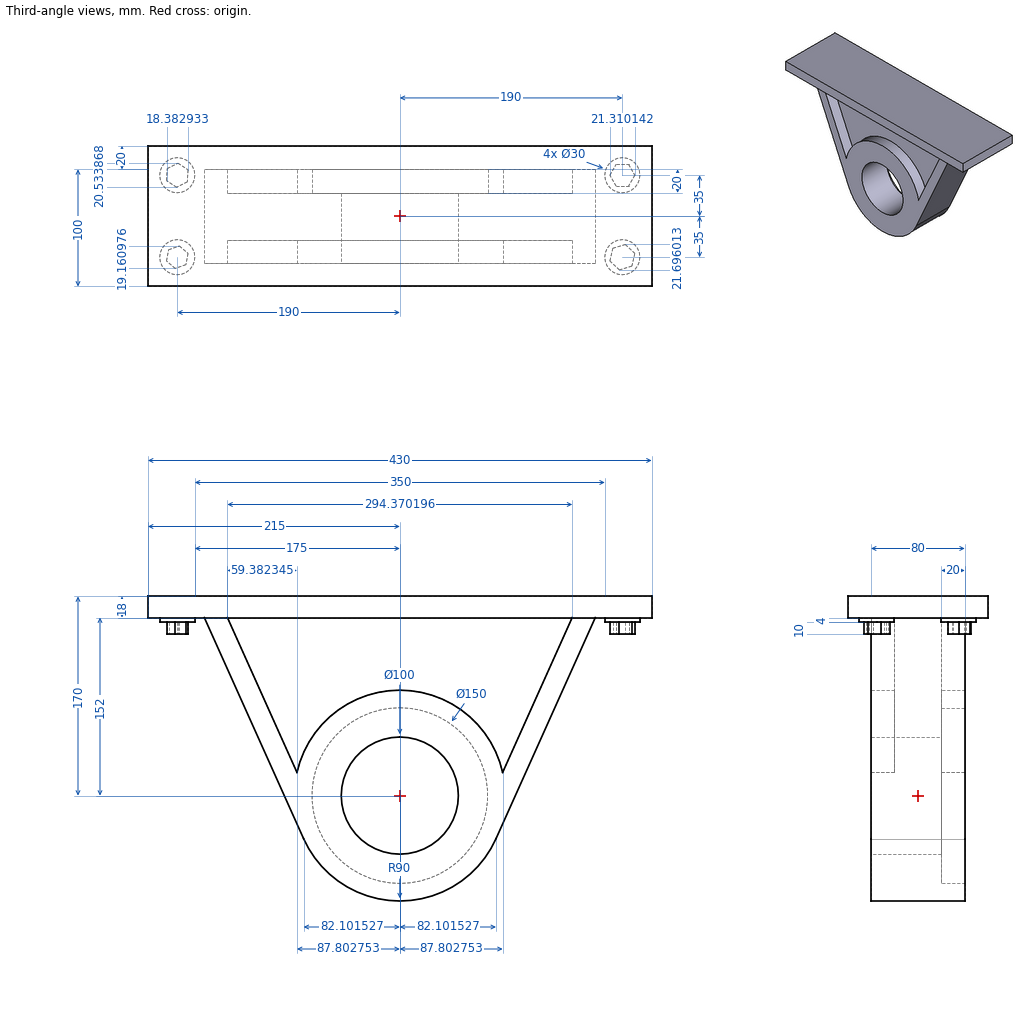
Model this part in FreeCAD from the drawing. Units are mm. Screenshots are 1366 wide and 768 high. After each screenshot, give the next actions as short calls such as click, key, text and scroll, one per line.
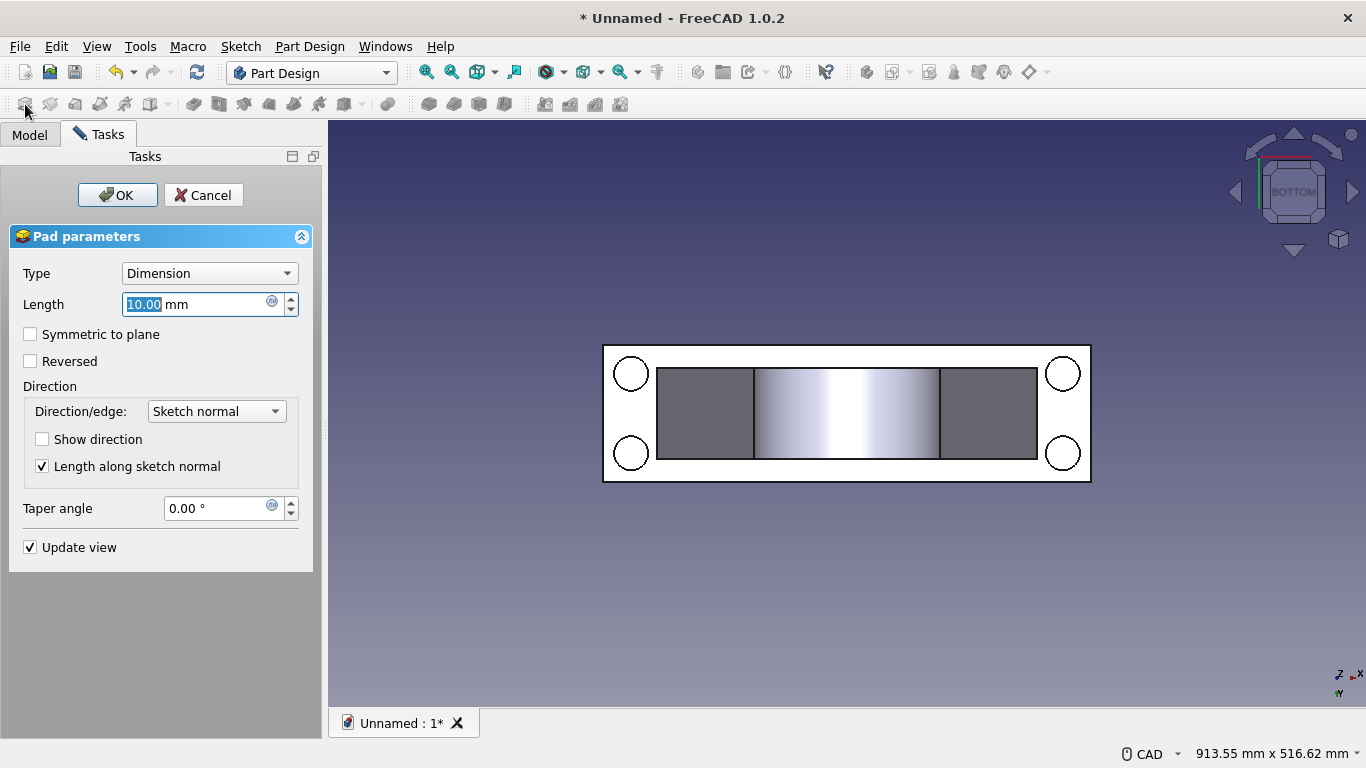
text(4)
key(Tab)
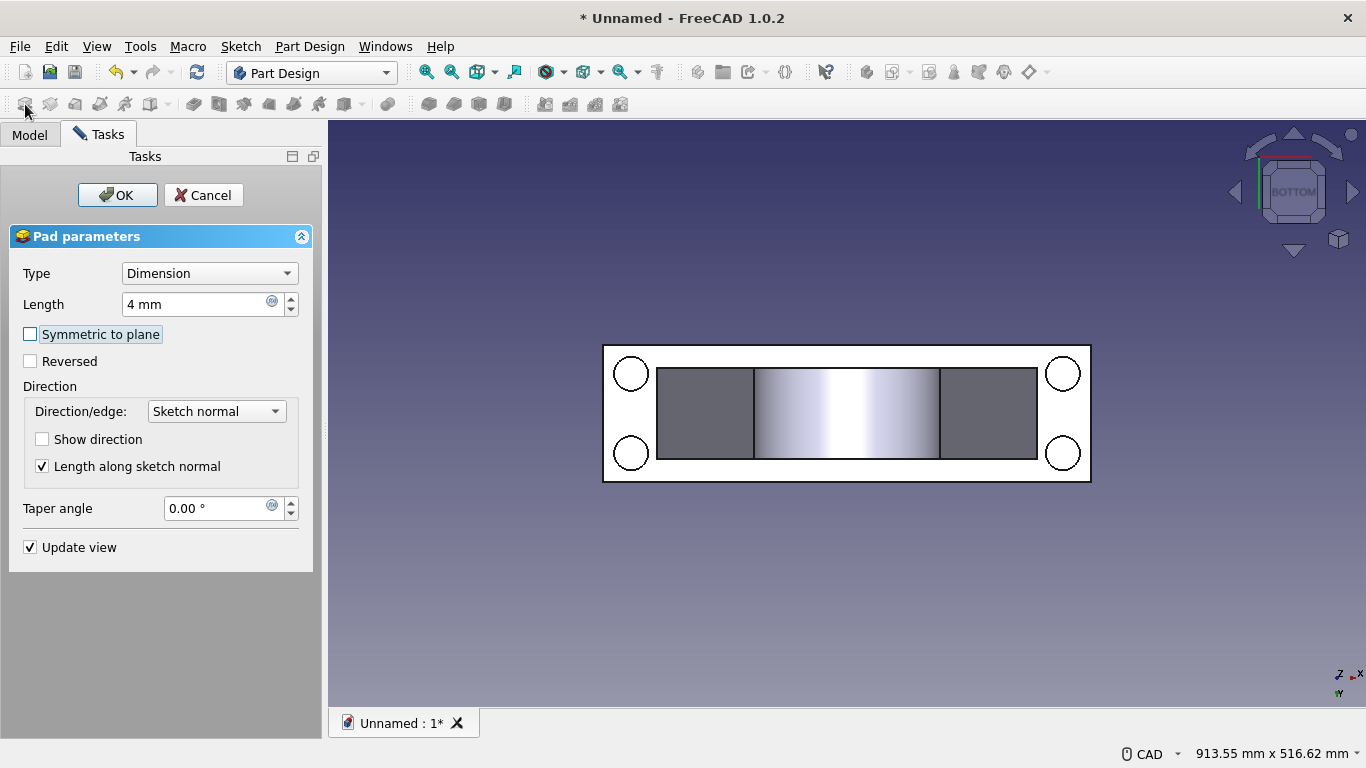
click(118, 195)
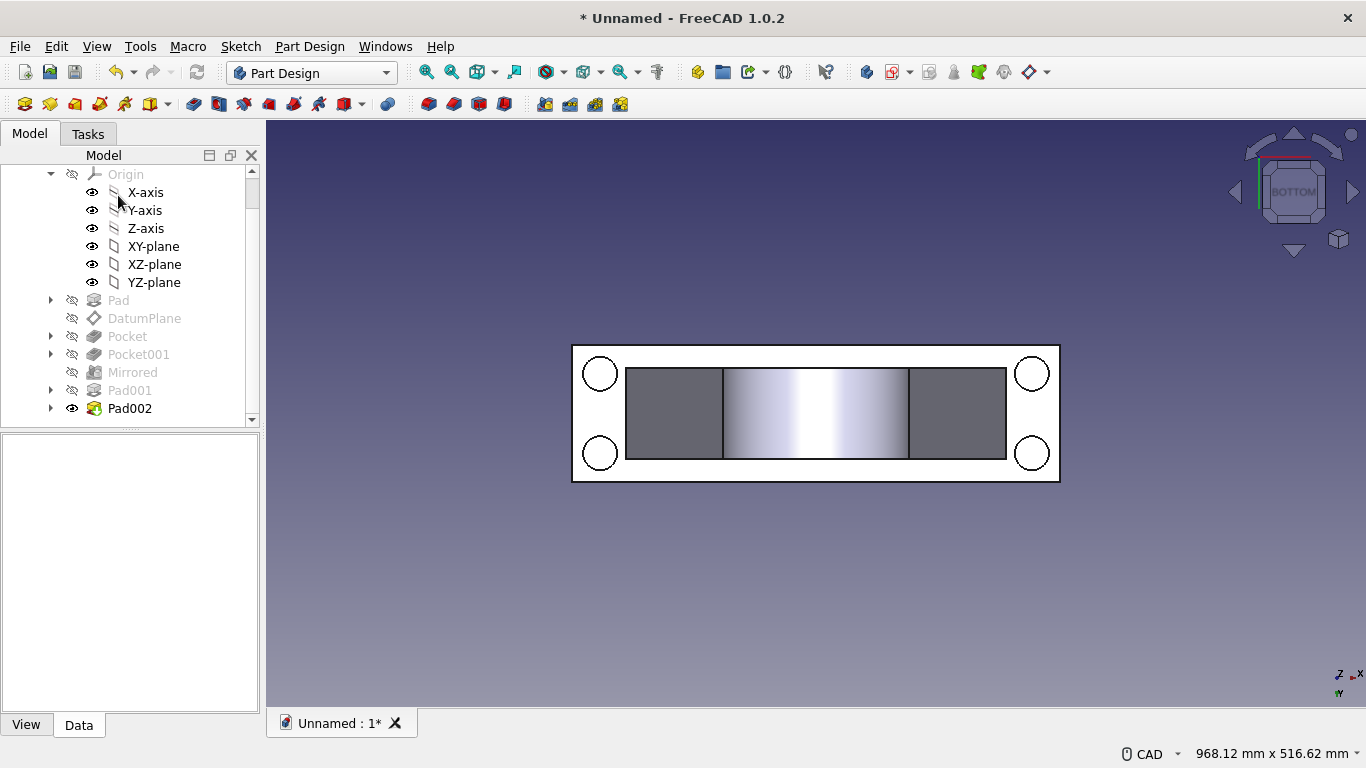
click(427, 72)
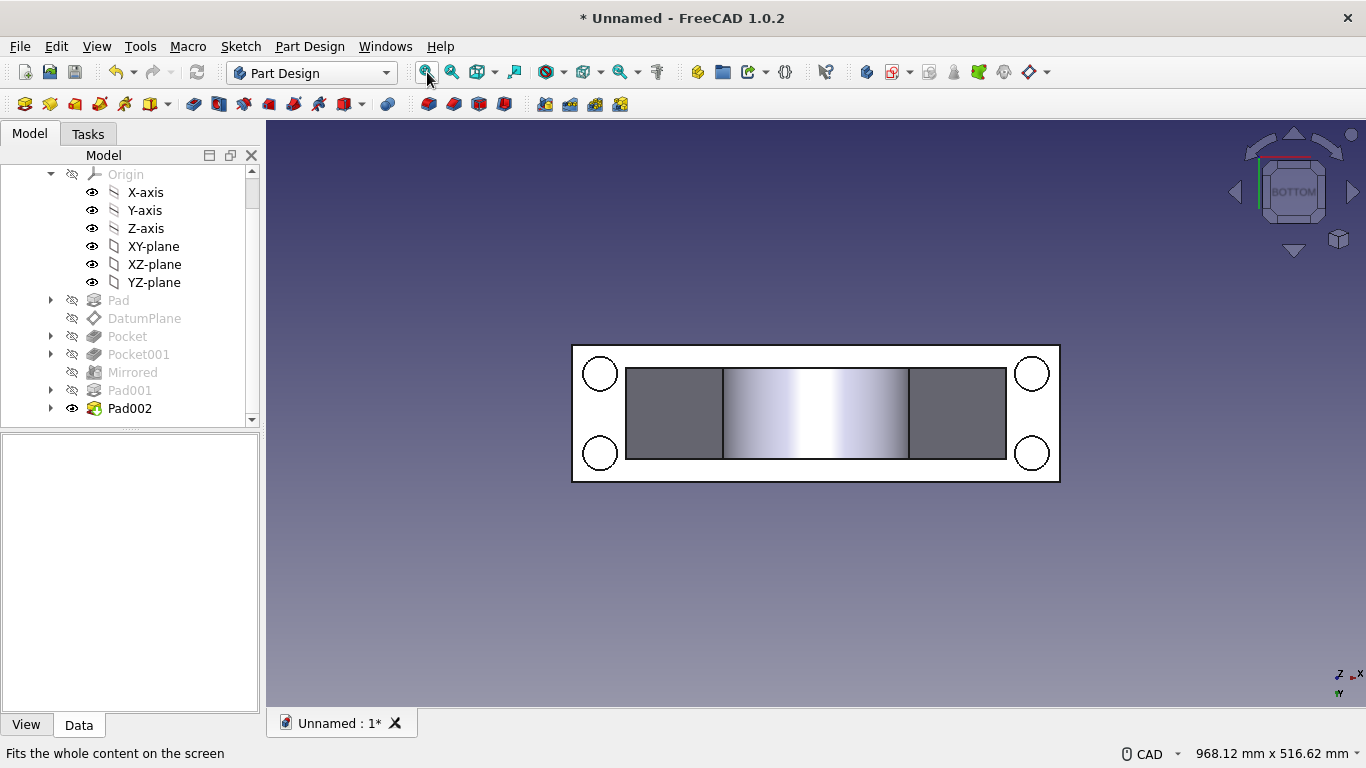
click(1032, 452)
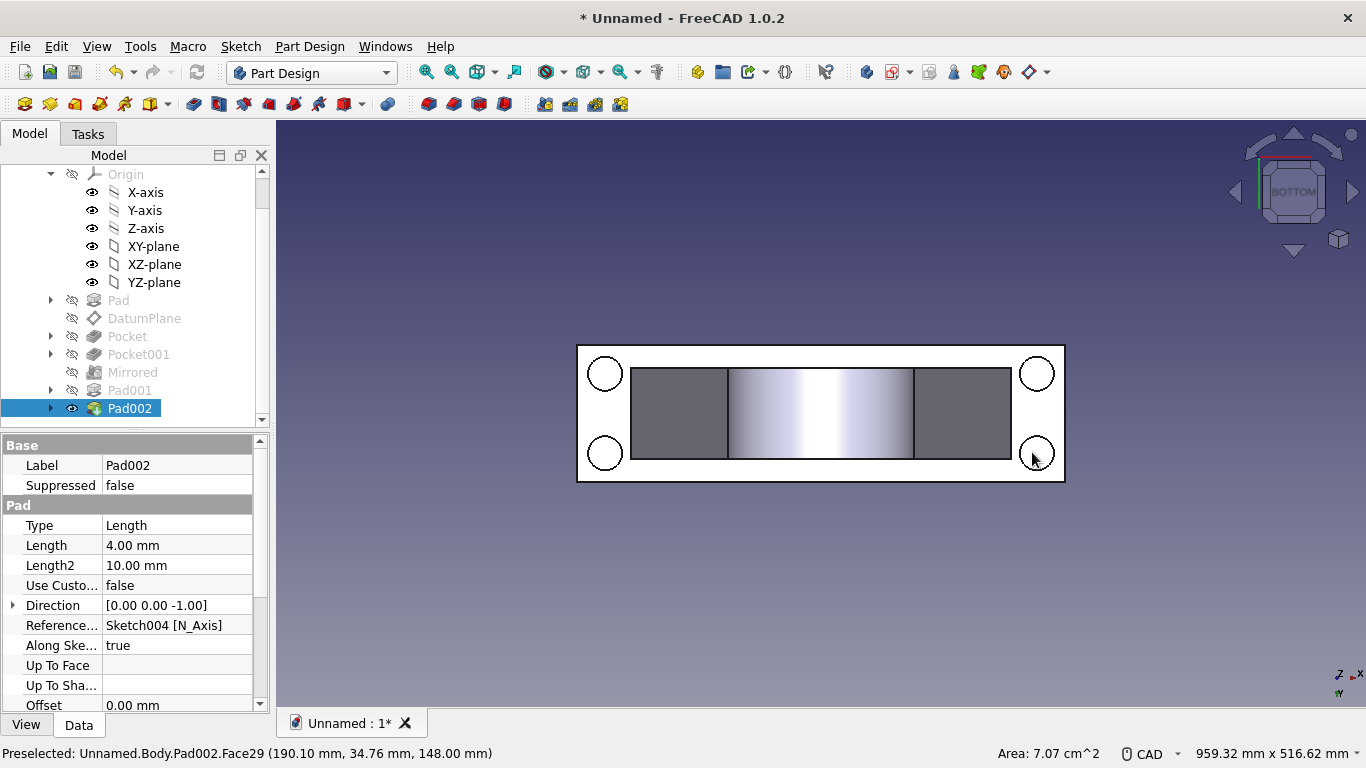
click(892, 72)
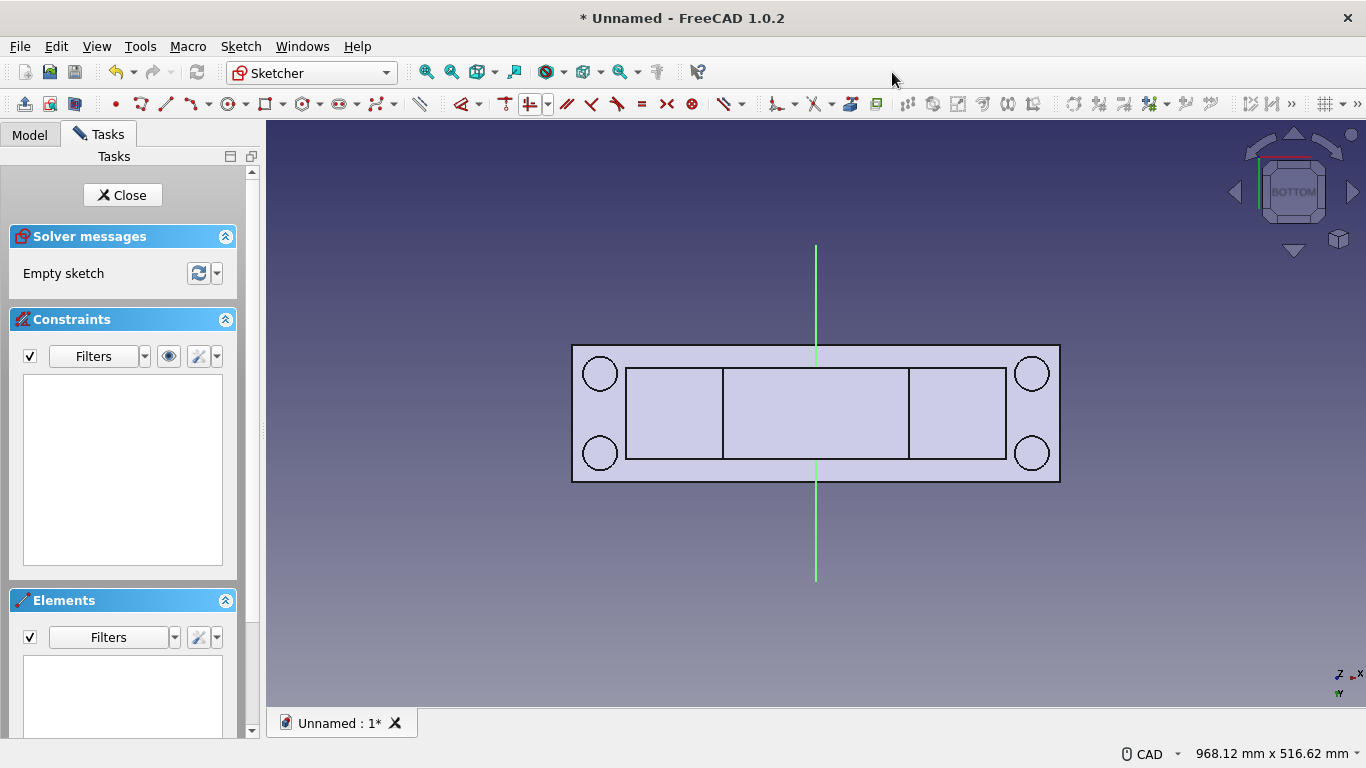
click(75, 104)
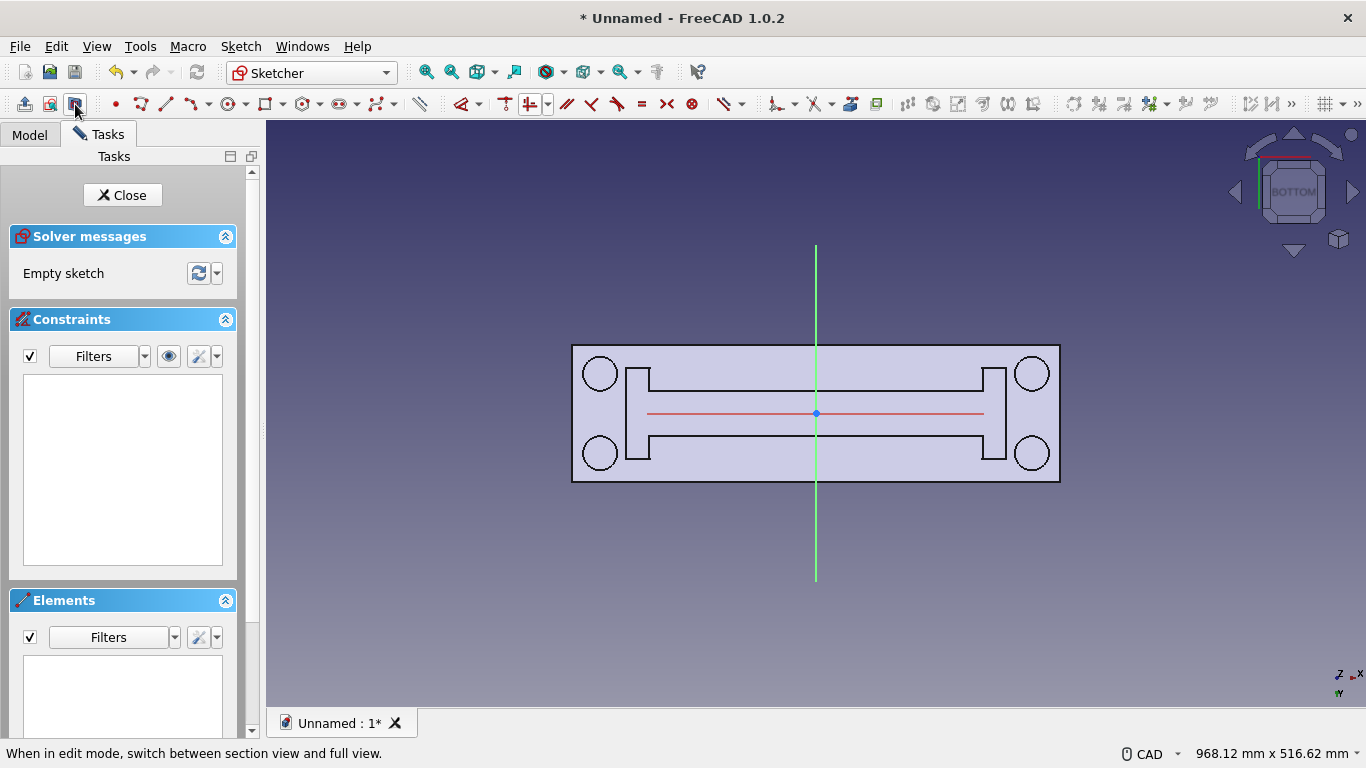
scroll(958, 412, up, 2)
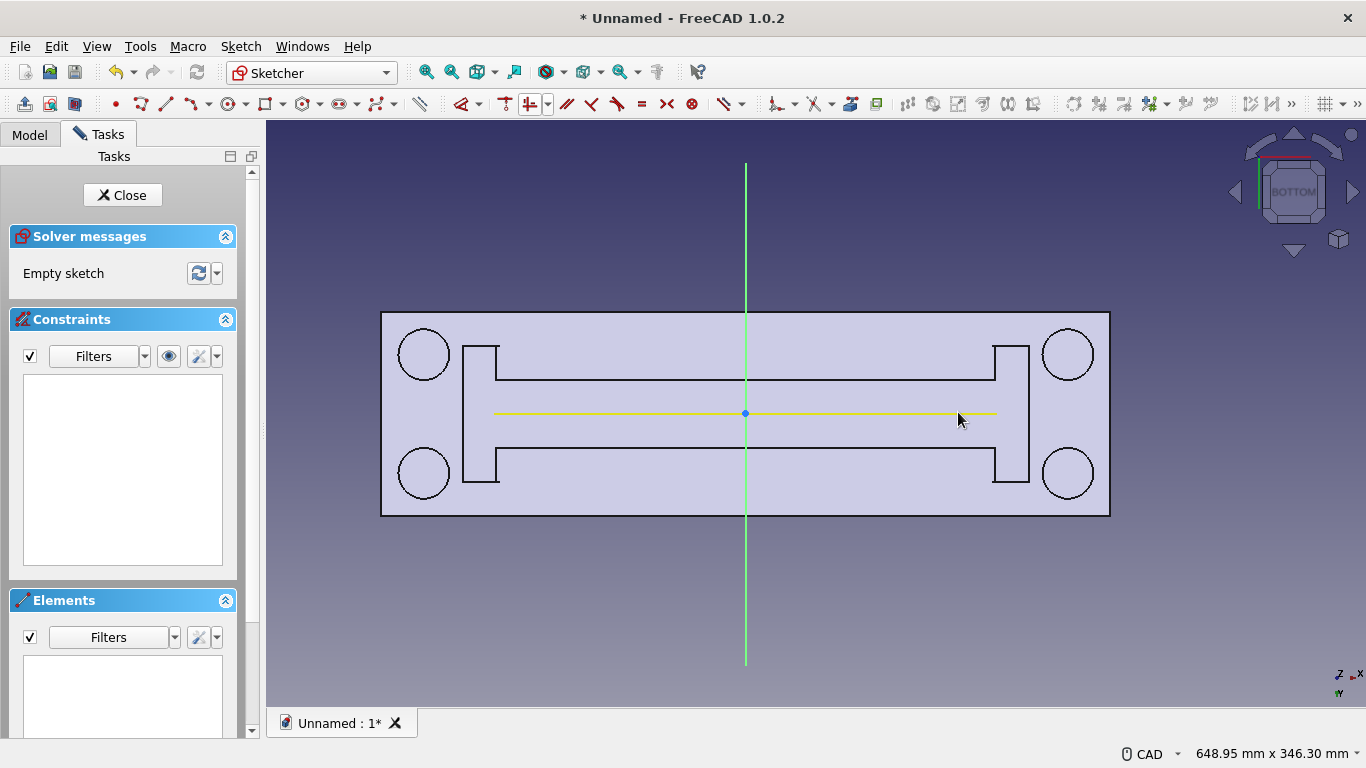
click(302, 104)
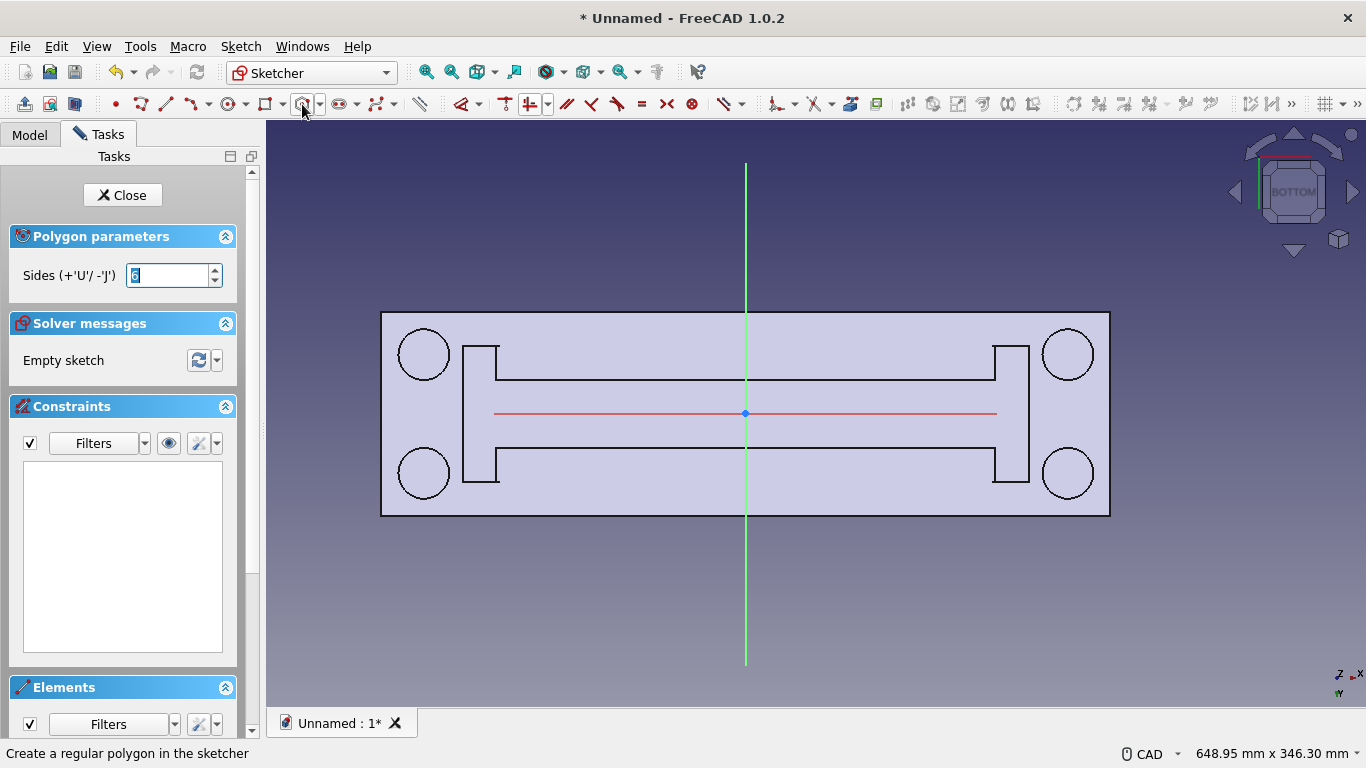
scroll(1068, 473, up, 3)